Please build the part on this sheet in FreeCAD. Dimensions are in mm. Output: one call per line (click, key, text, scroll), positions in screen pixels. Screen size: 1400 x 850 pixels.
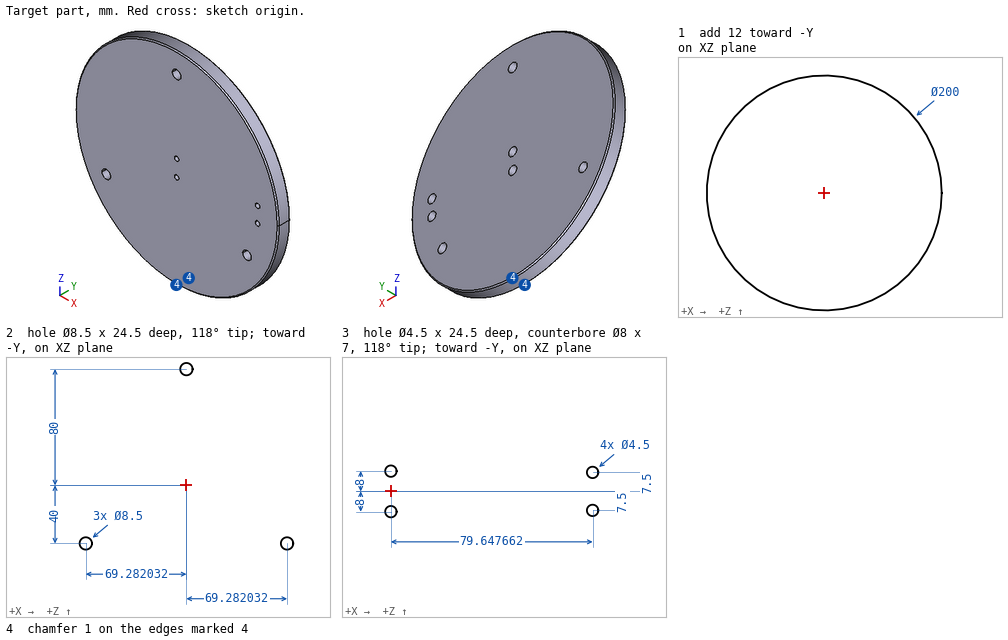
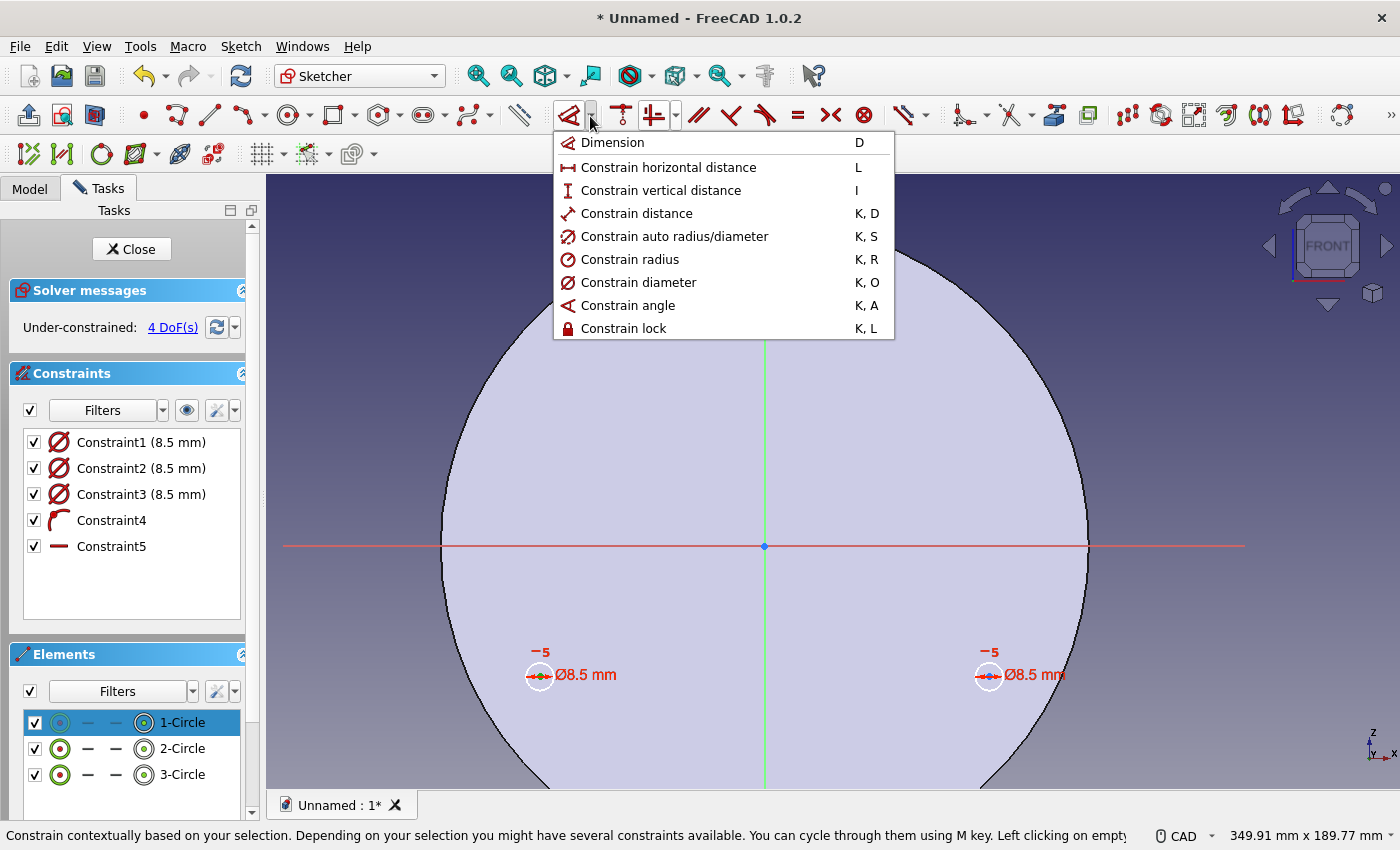
click(724, 190)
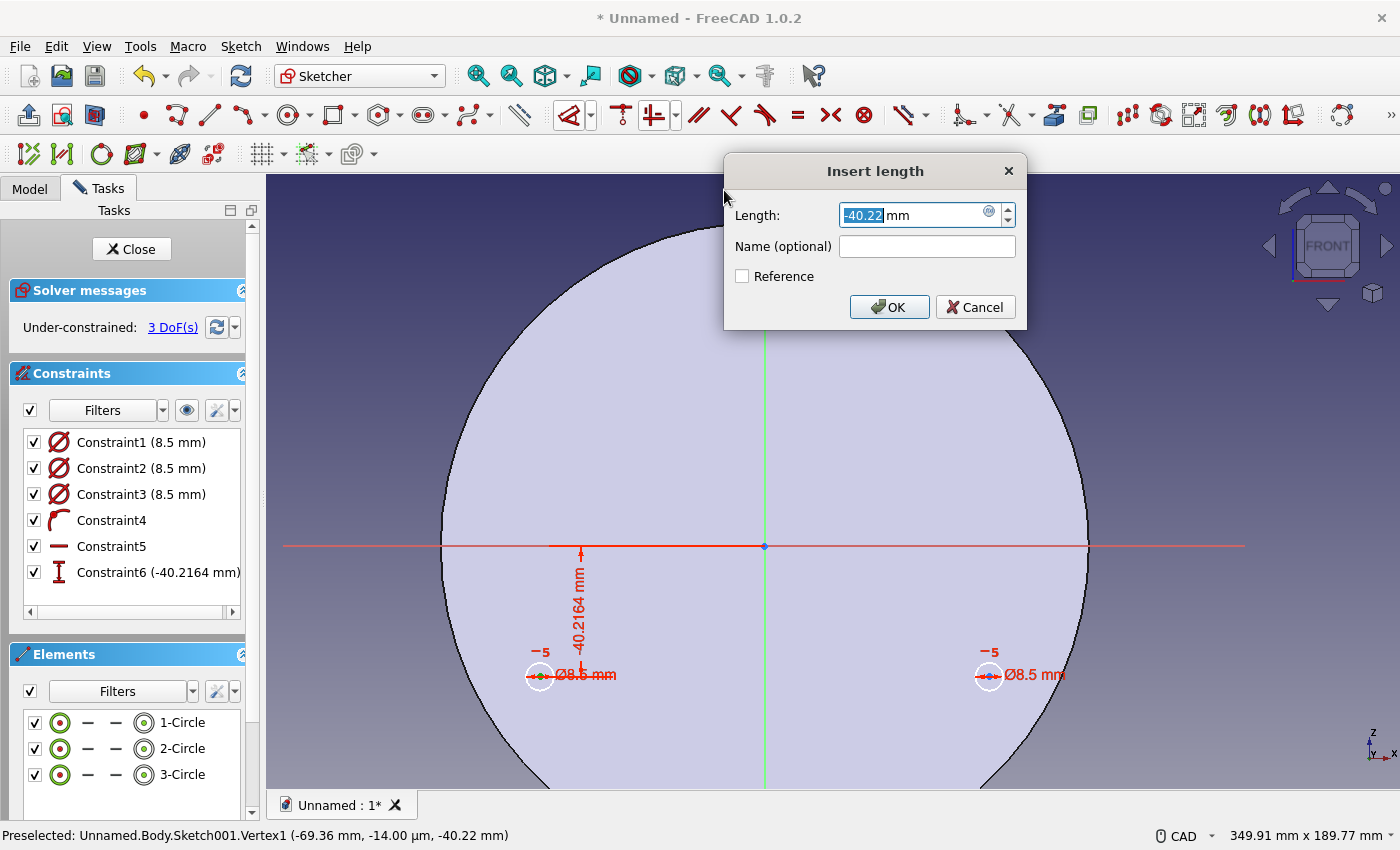
text(-40)
key(Return)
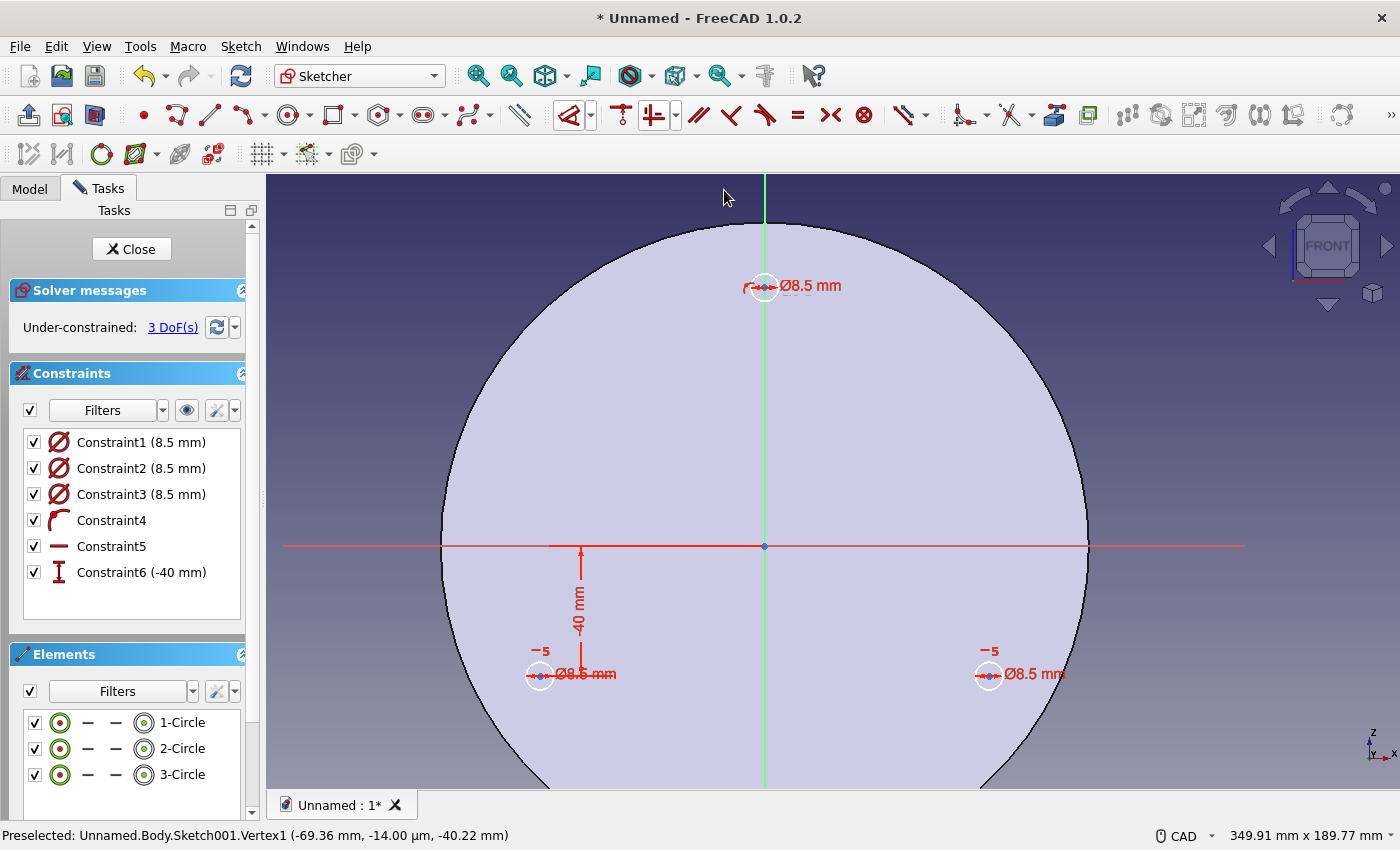
click(765, 288)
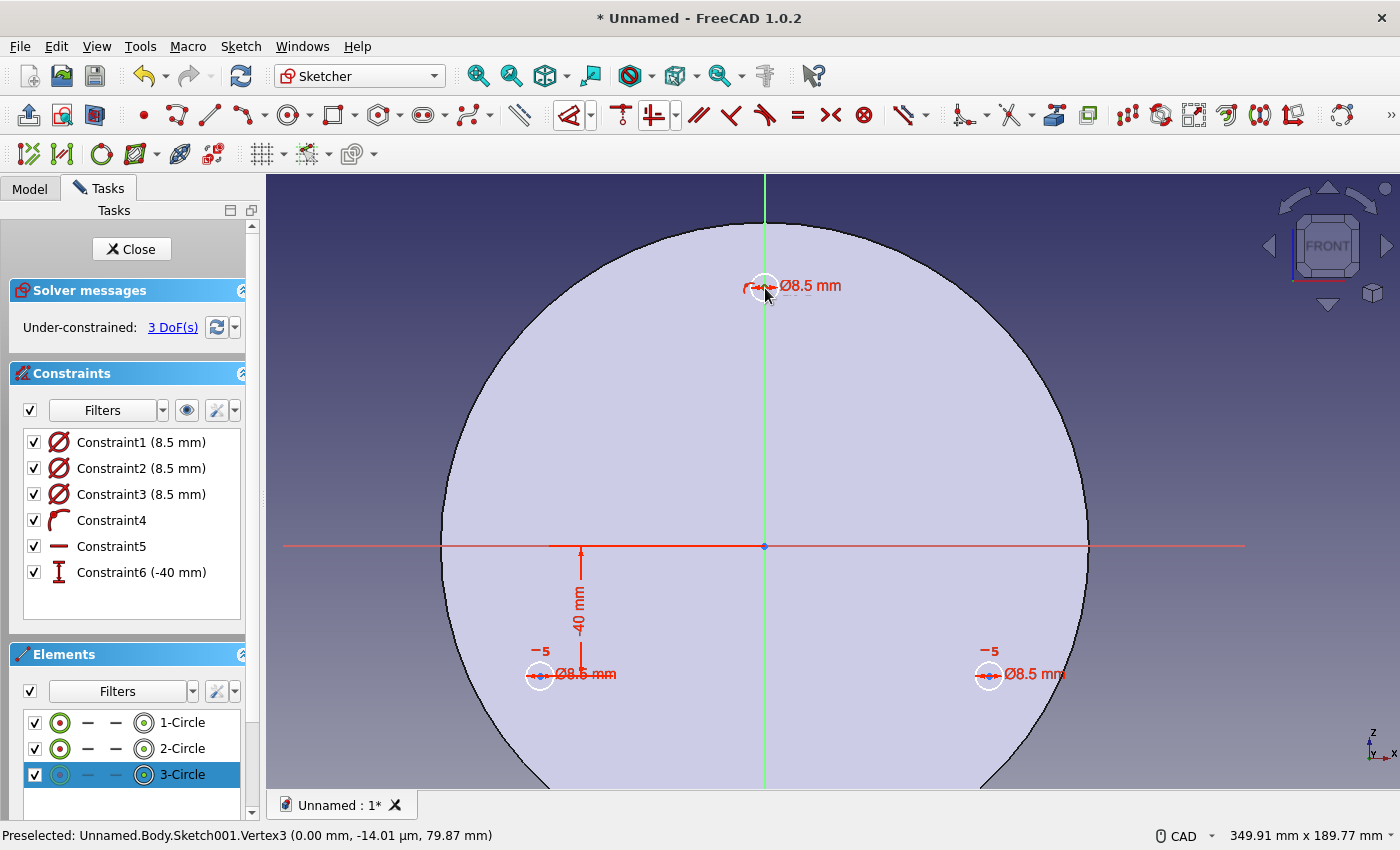
key(i)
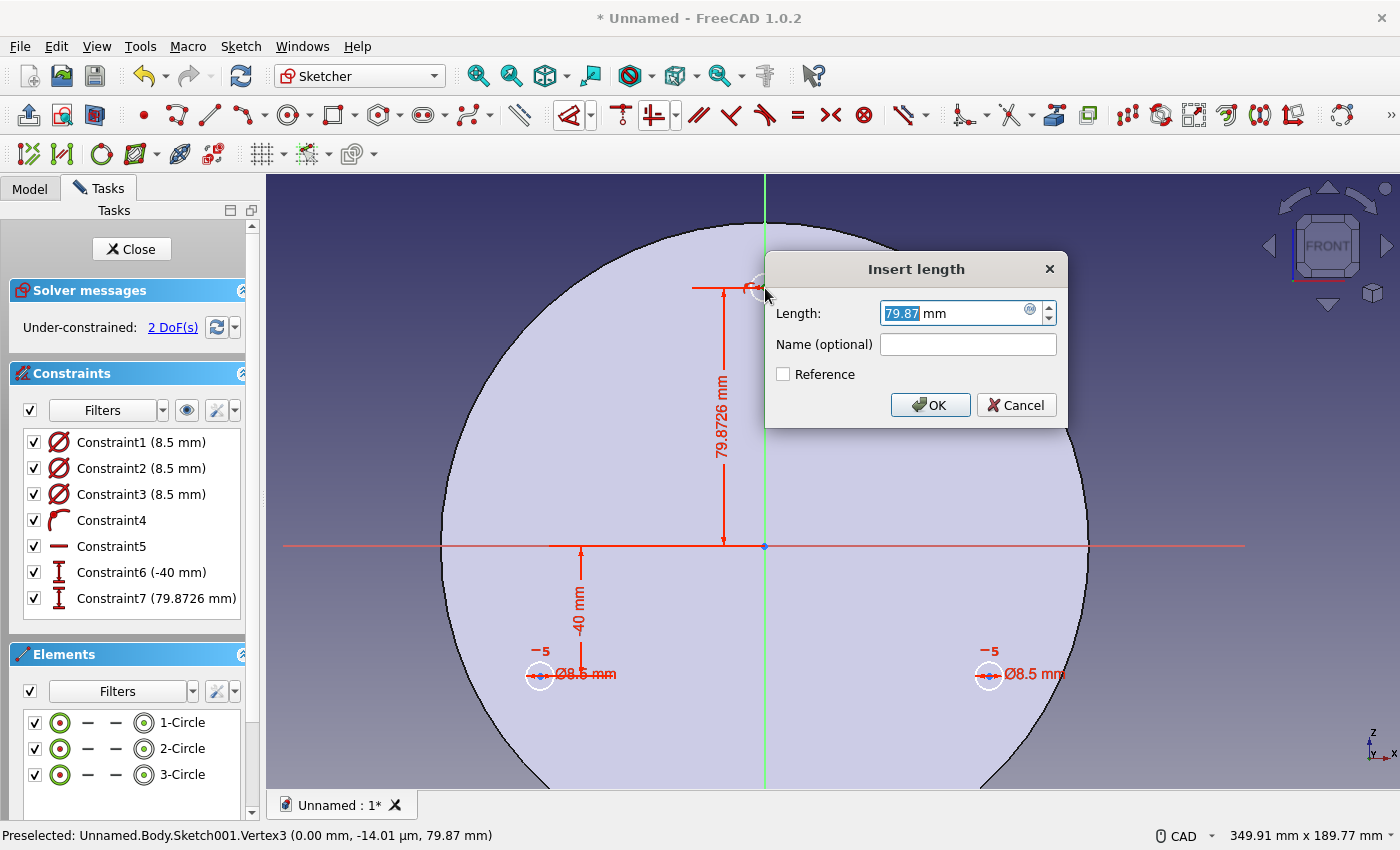
text(80)
key(Return)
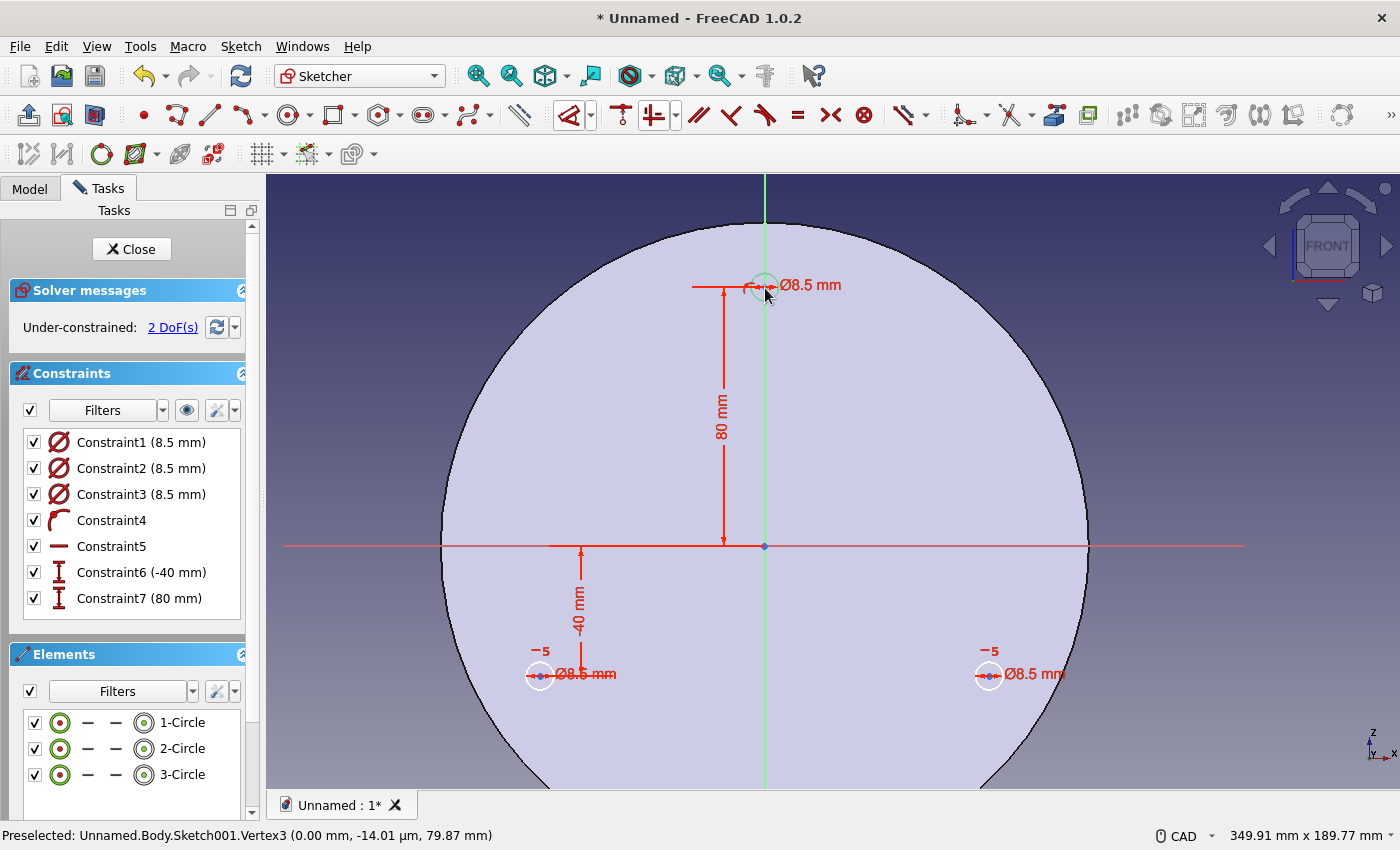
click(540, 676)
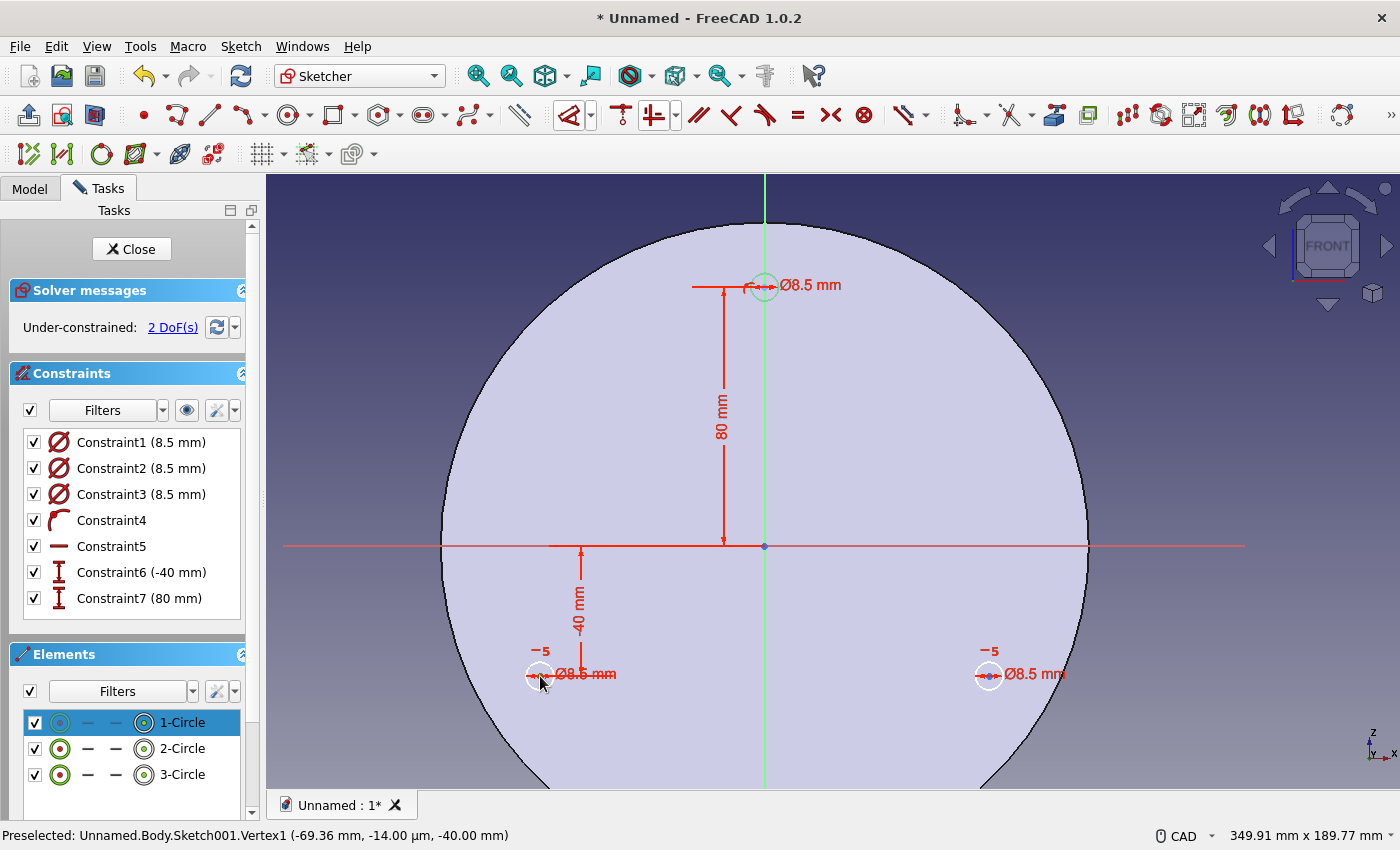
key(l)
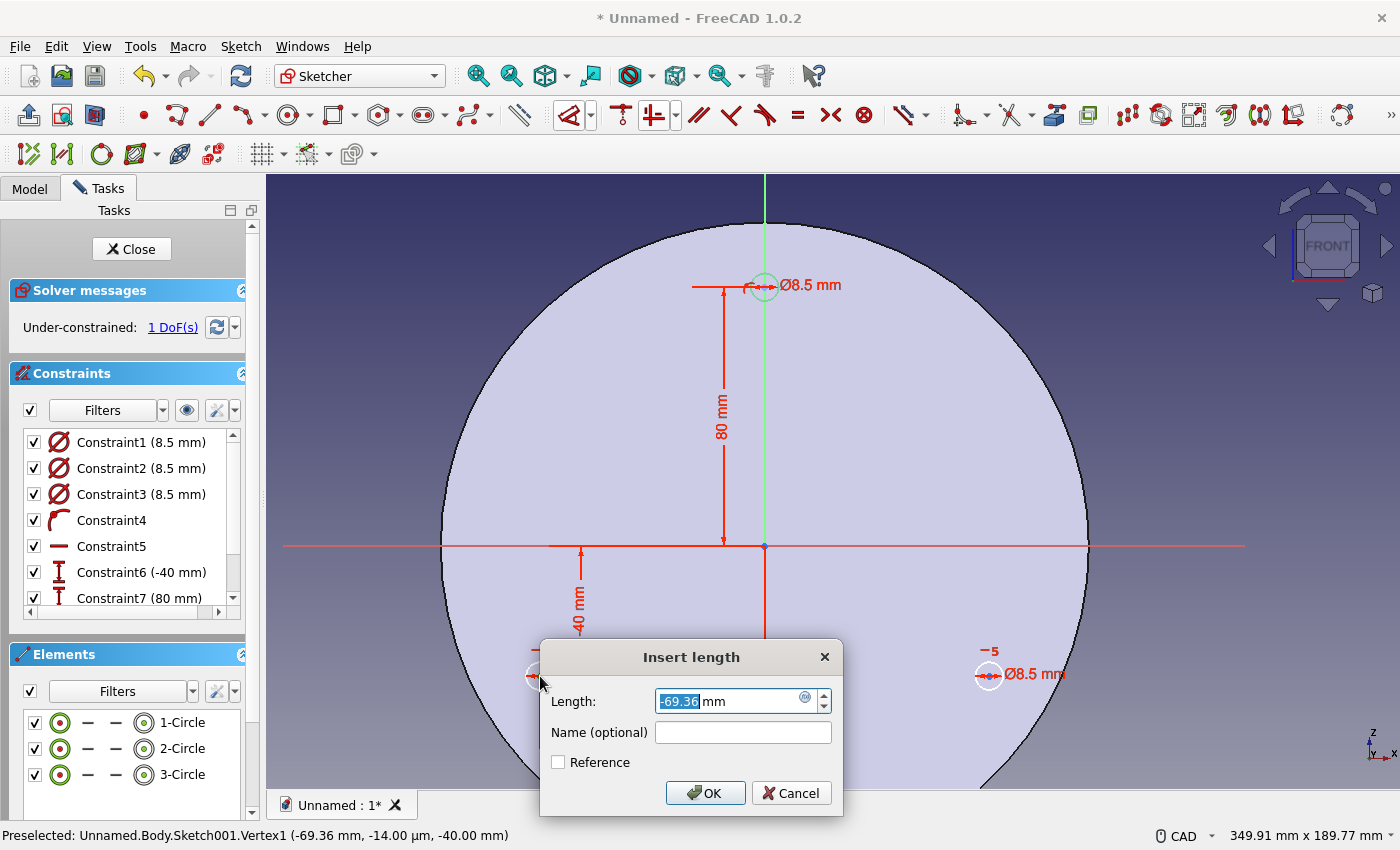
text(-69.282032)
key(Return)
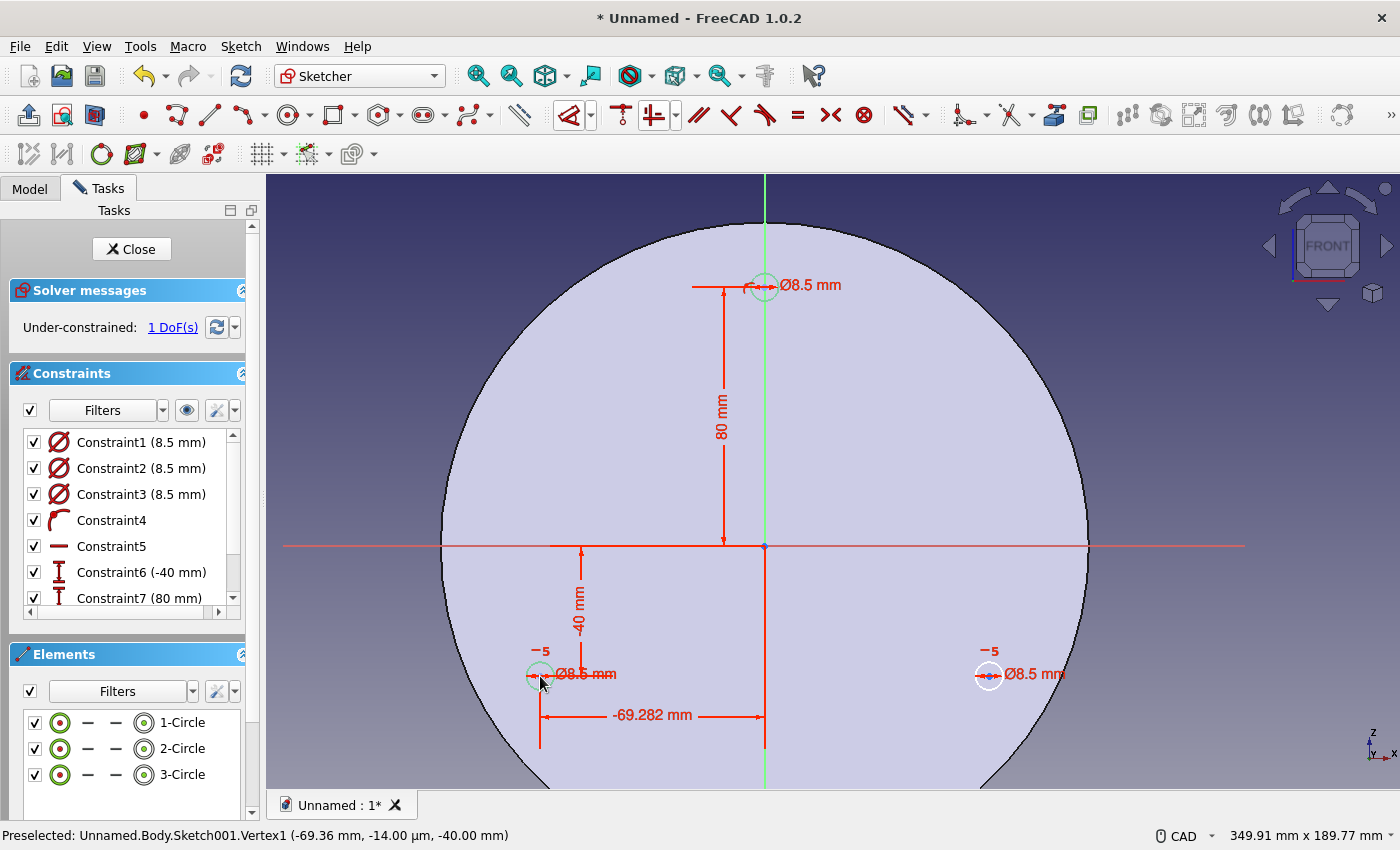
click(989, 676)